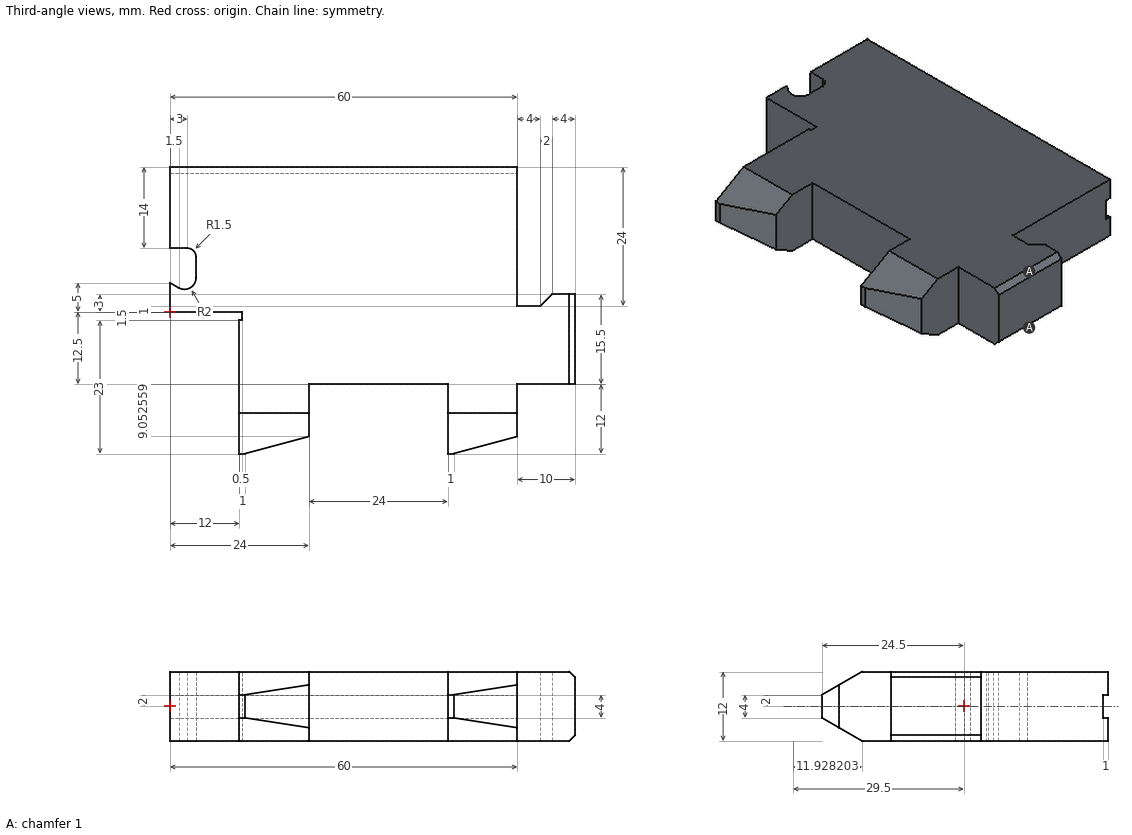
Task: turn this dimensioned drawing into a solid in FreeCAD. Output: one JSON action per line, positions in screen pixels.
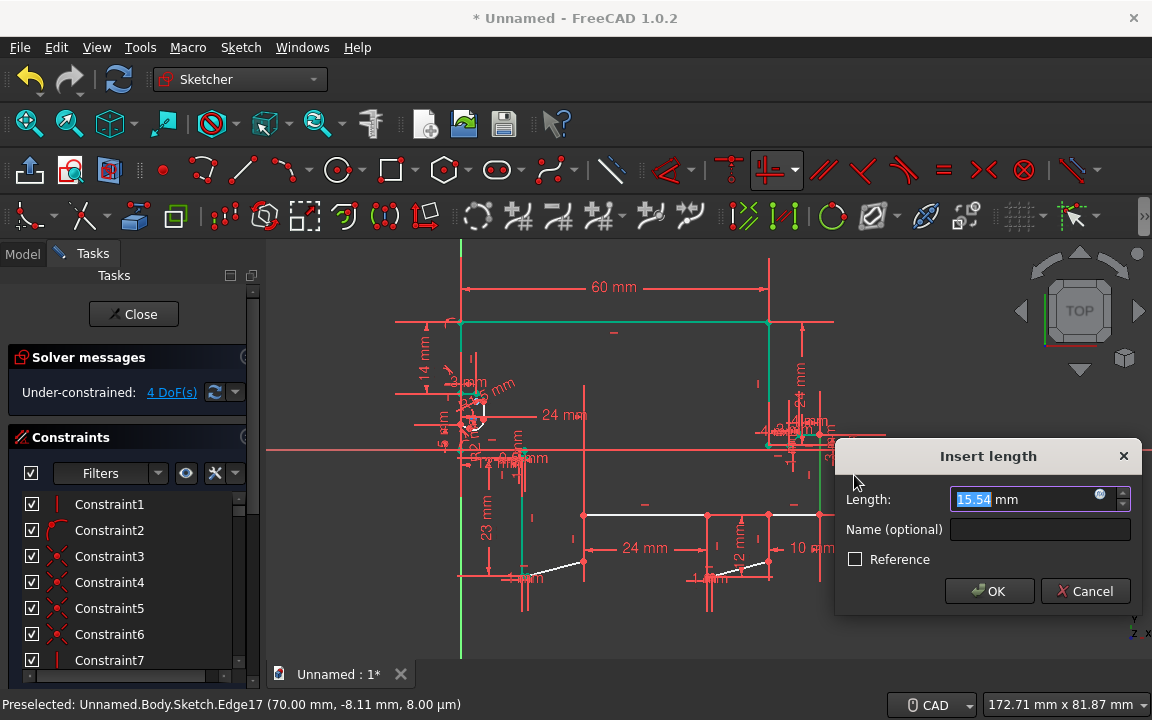
{"action": "type", "text": "15.5"}
{"action": "key", "text": "Return"}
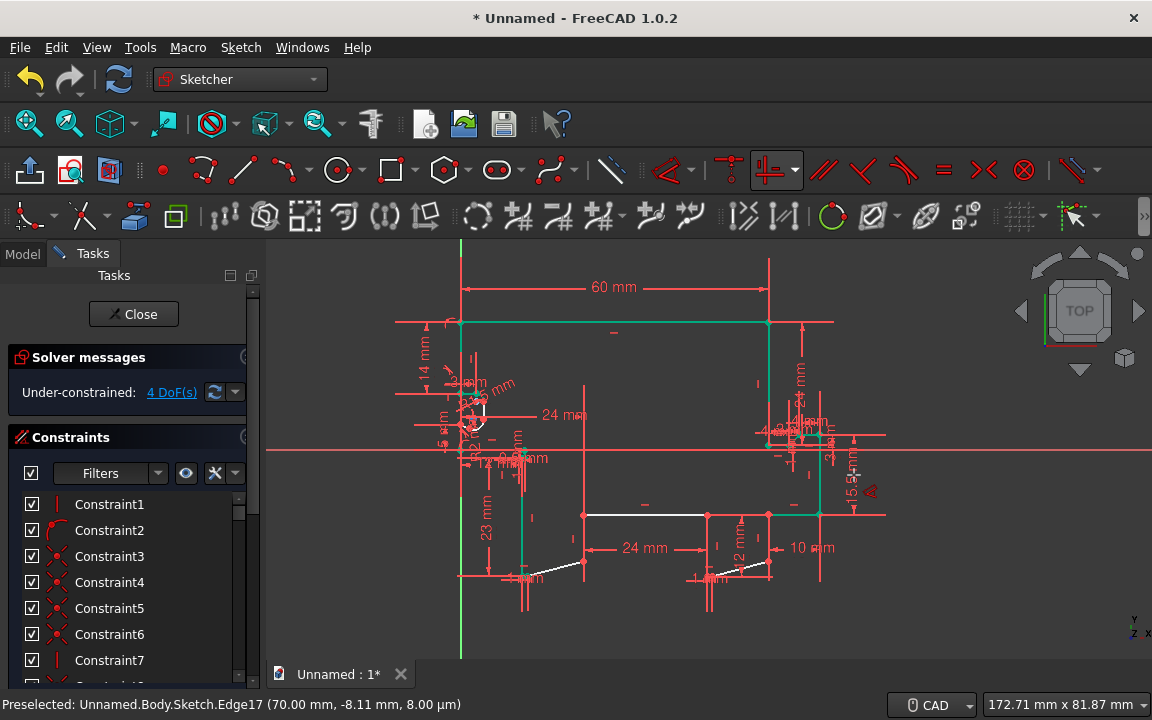
{"action": "scroll", "coordinate": [469, 429], "scroll_direction": "up", "scroll_amount": 9}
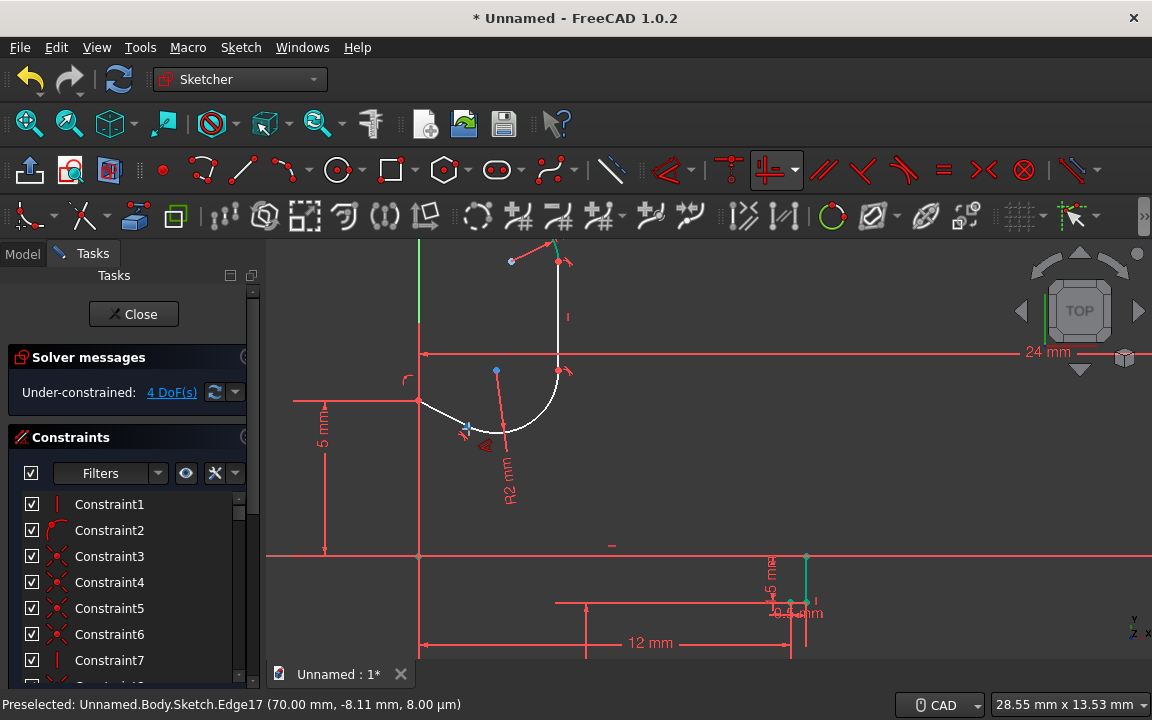
{"action": "left_click", "coordinate": [468, 426]}
{"action": "left_click", "coordinate": [443, 392]}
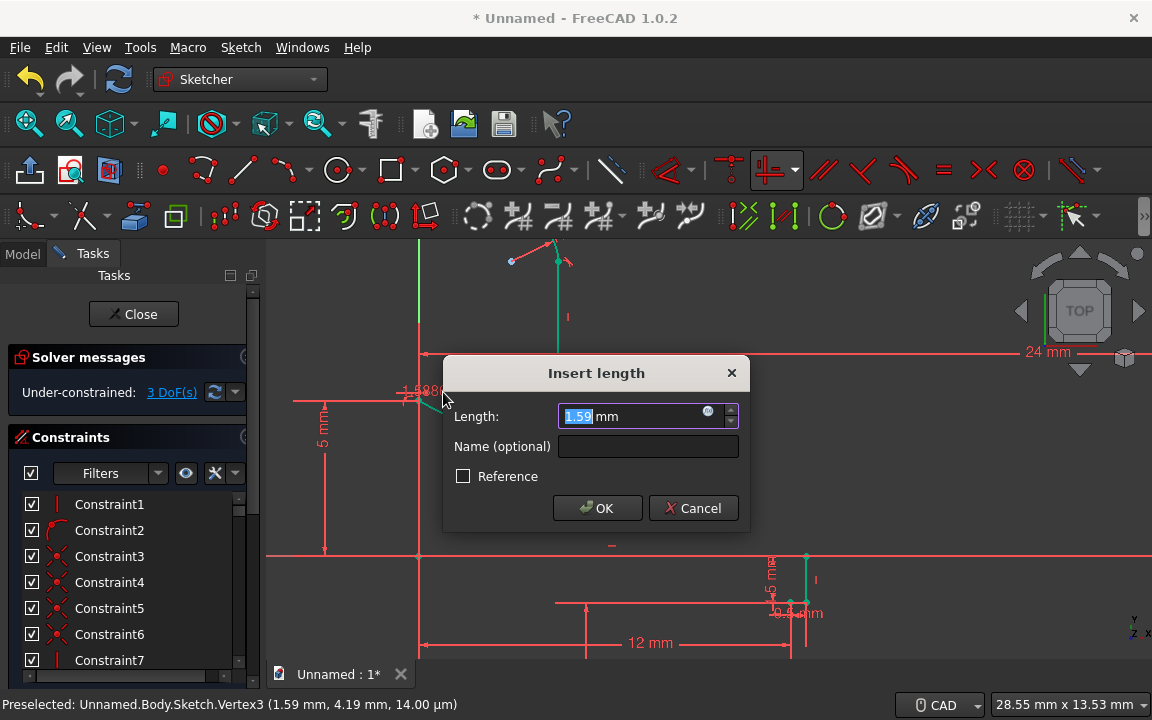
{"action": "type", "text": "1.5"}
{"action": "key", "text": "Return"}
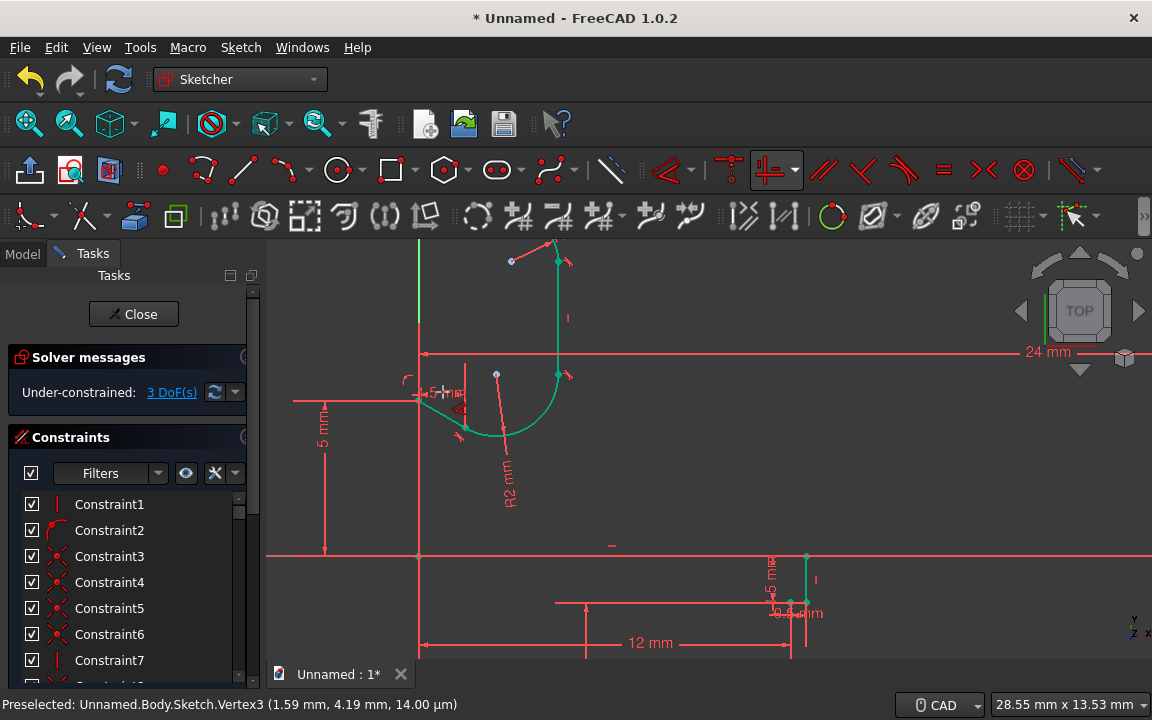
{"action": "scroll", "coordinate": [469, 429], "scroll_direction": "down", "scroll_amount": 9}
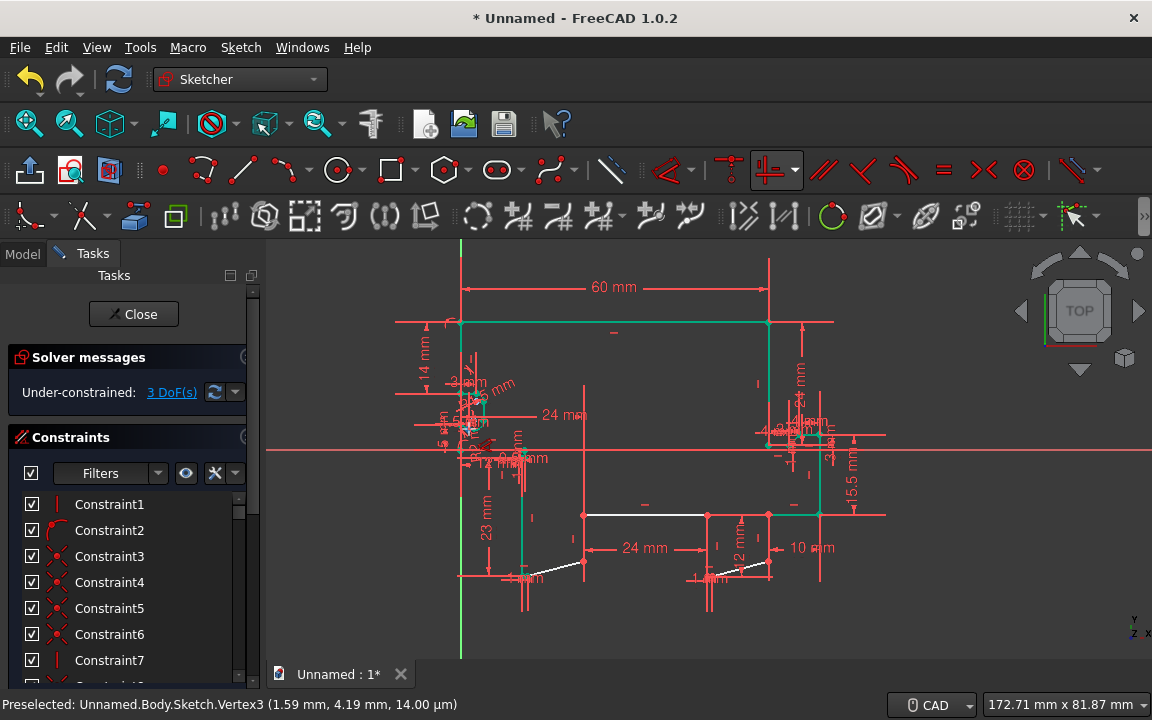
{"action": "left_click", "coordinate": [584, 515]}
{"action": "left_click", "coordinate": [427, 483]}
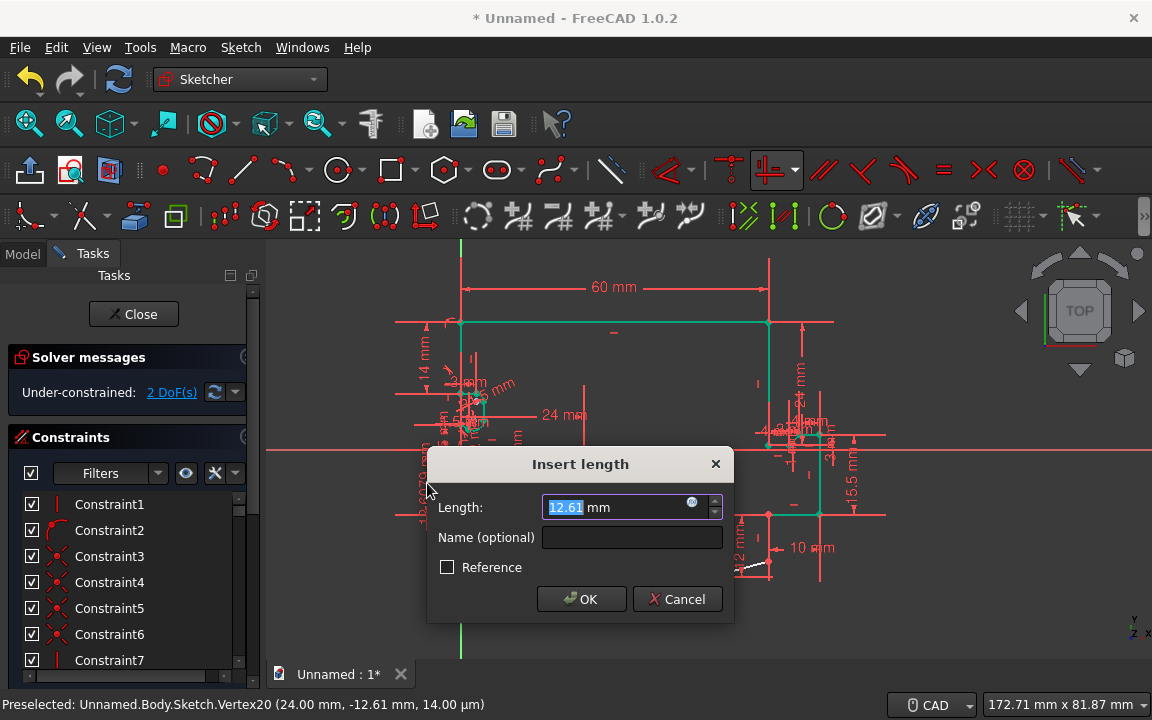
{"action": "type", "text": "12.5"}
{"action": "key", "text": "Return"}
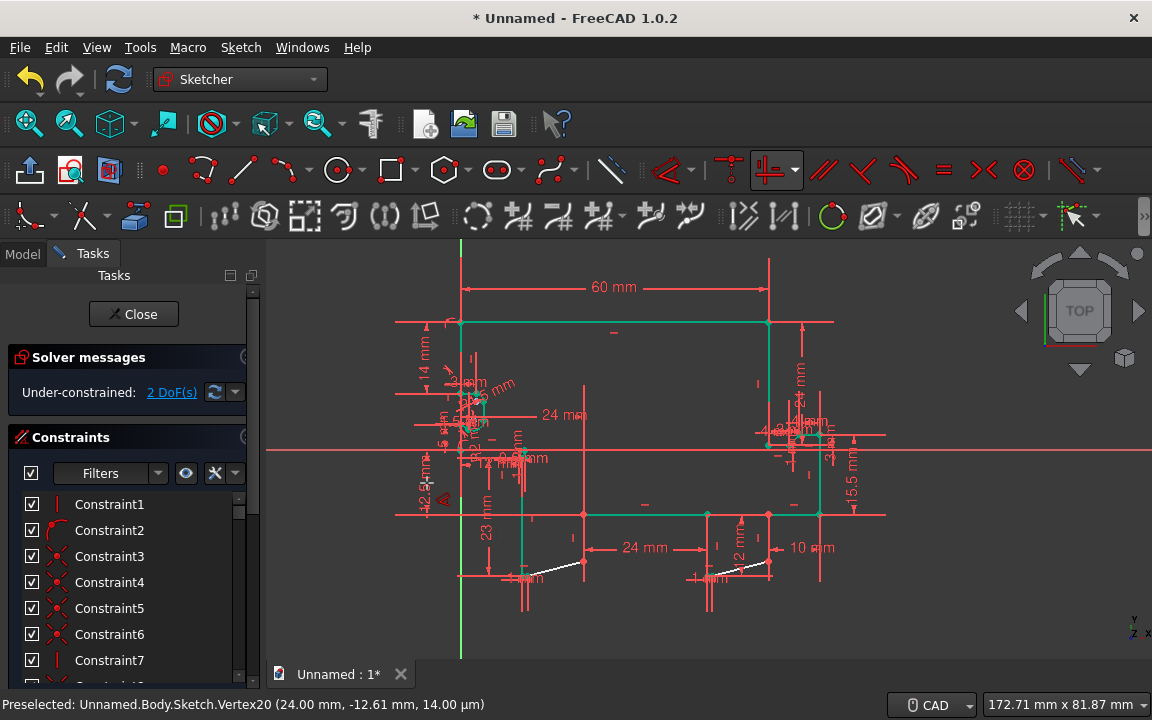
{"action": "left_click", "coordinate": [584, 547]}
{"action": "left_click", "coordinate": [550, 549]}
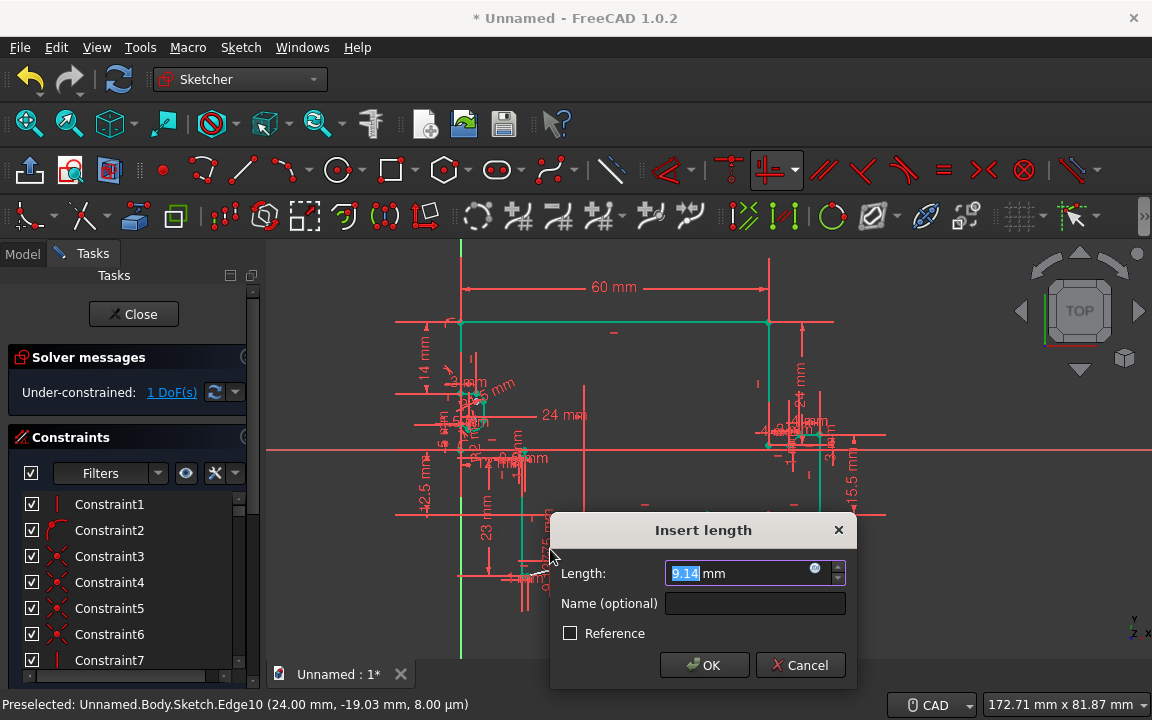
{"action": "type", "text": "9.052559"}
{"action": "key", "text": "Return"}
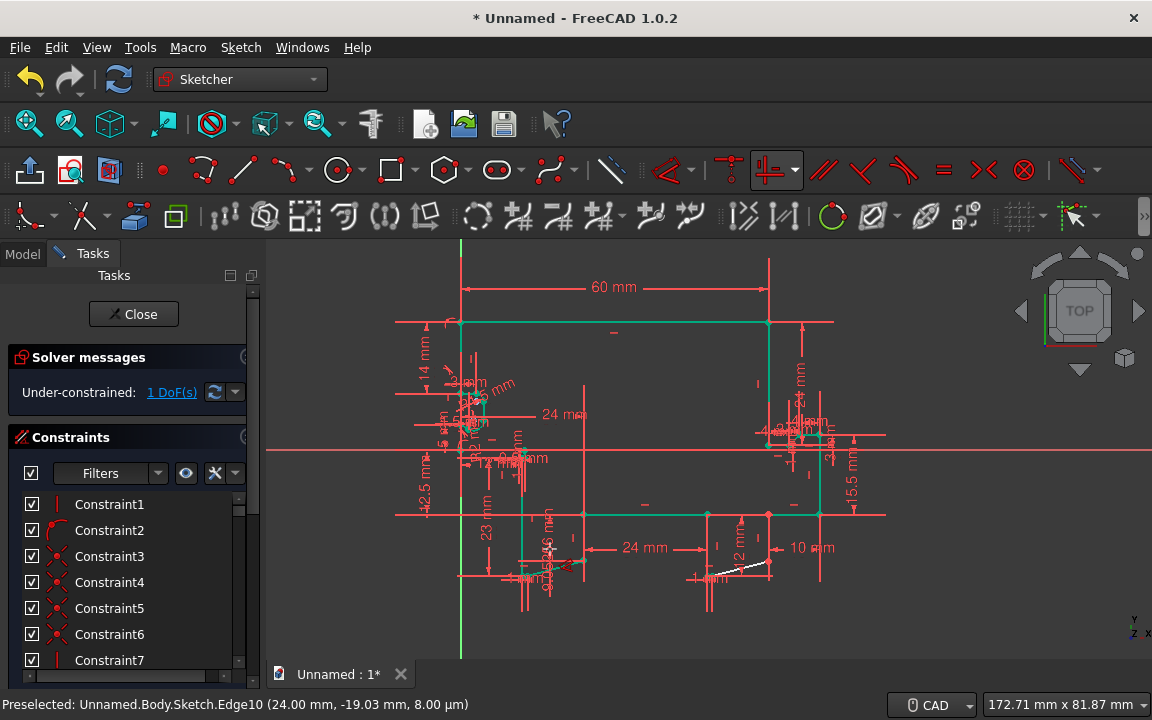
{"action": "left_click", "coordinate": [769, 547]}
{"action": "left_click", "coordinate": [735, 522]}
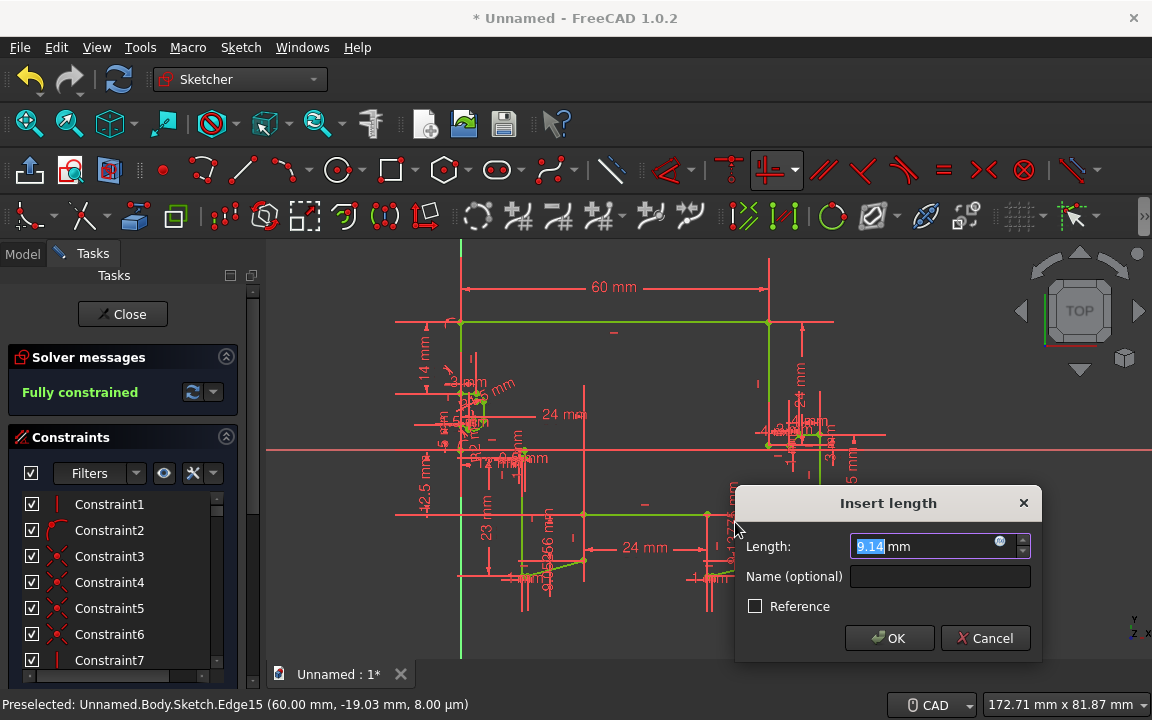
{"action": "type", "text": "9.052559"}
{"action": "key", "text": "Return"}
{"action": "key", "text": "Escape"}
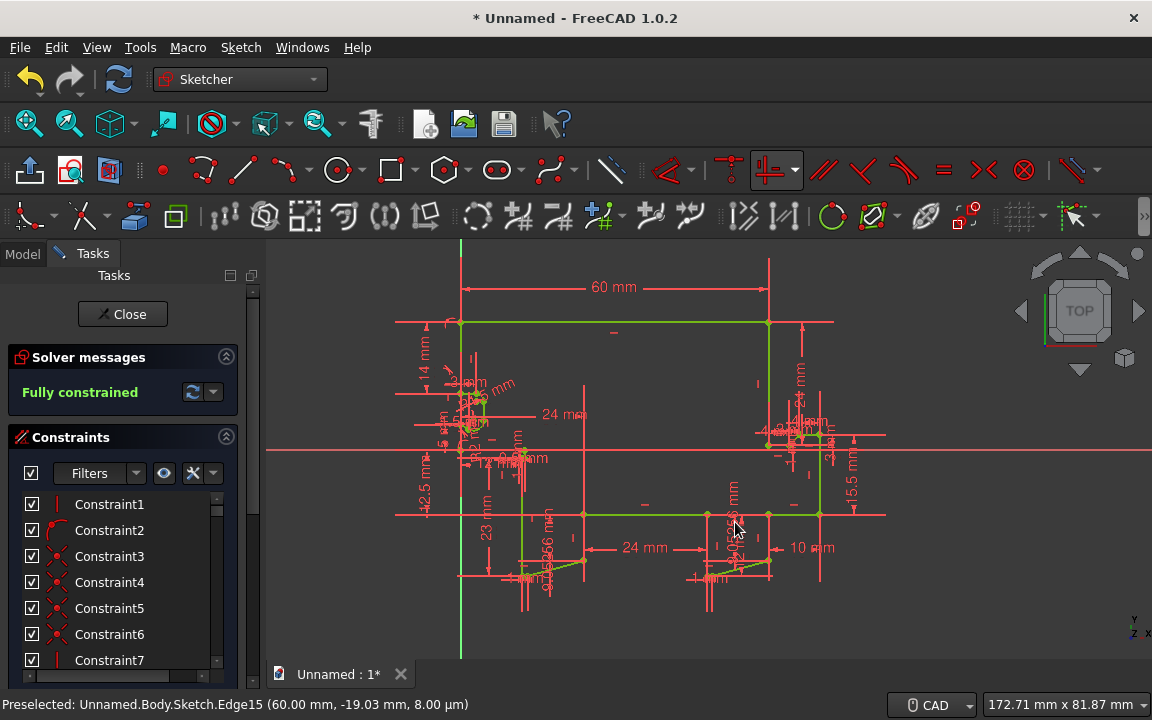
{"action": "left_click", "coordinate": [123, 314]}